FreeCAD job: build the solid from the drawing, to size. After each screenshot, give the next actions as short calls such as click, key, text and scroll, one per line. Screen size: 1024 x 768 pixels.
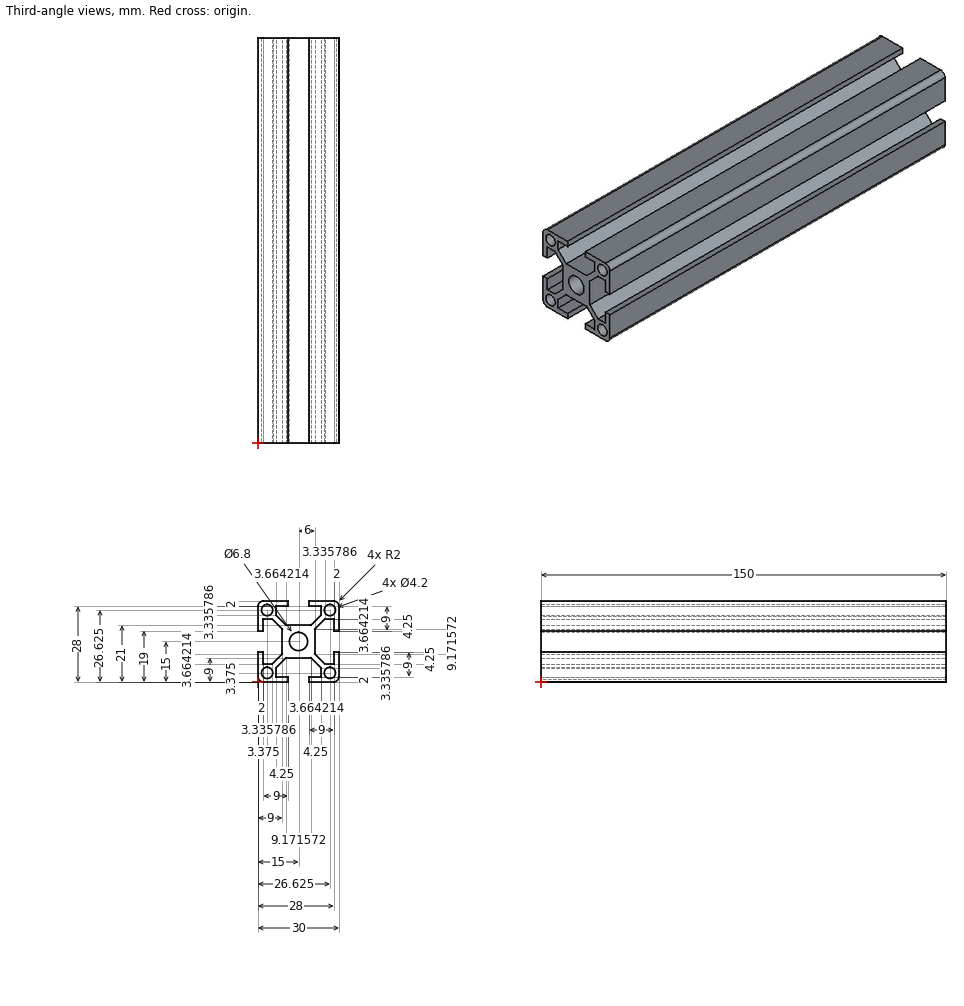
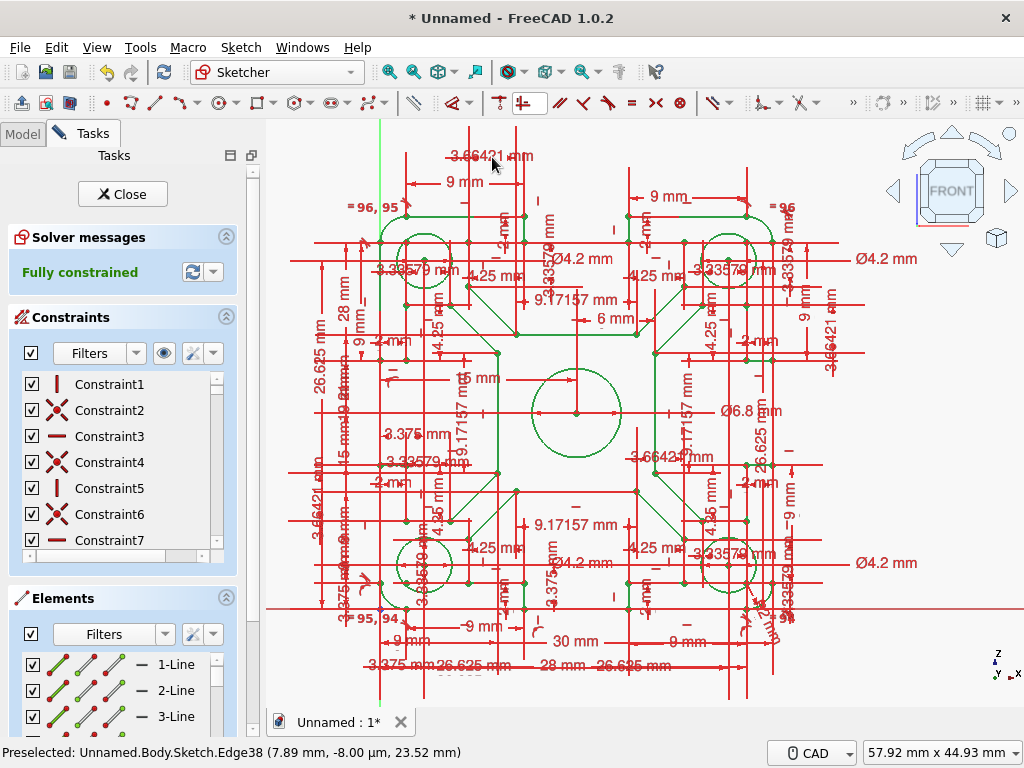
click(123, 194)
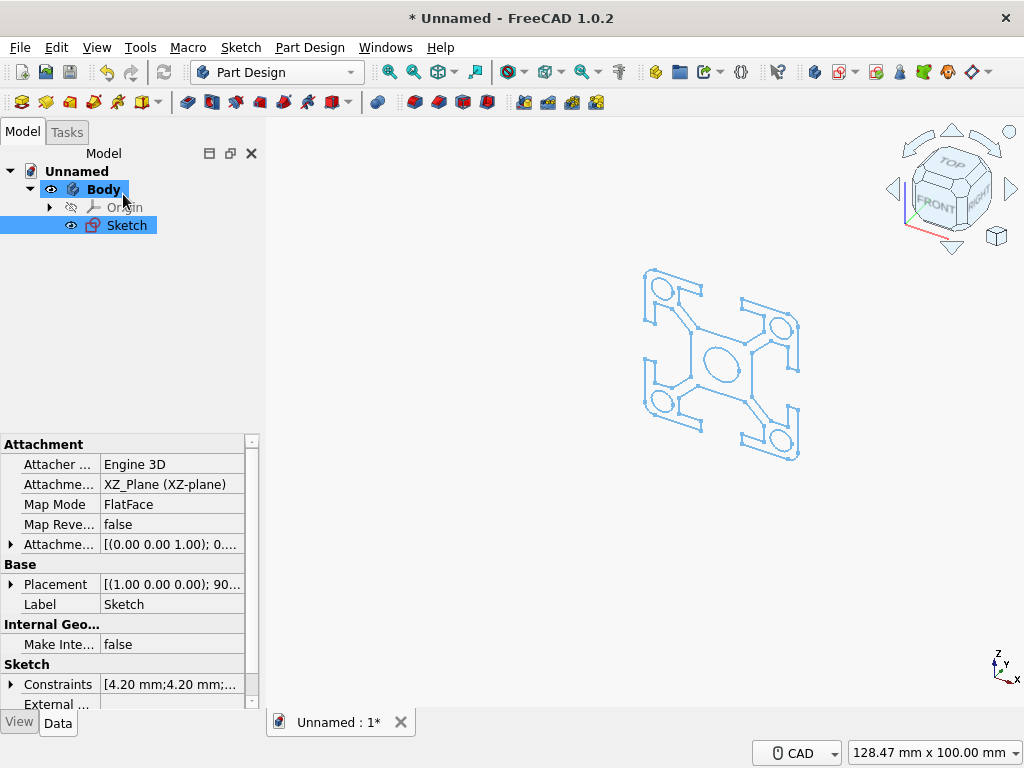
click(22, 102)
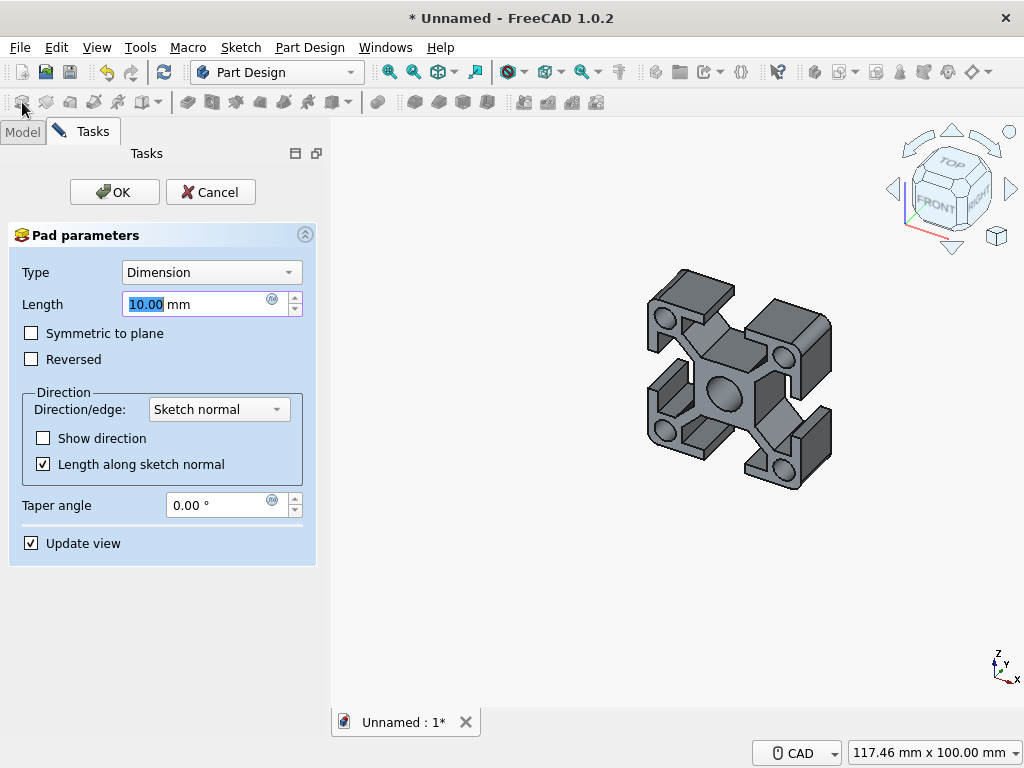
text(150)
key(Tab)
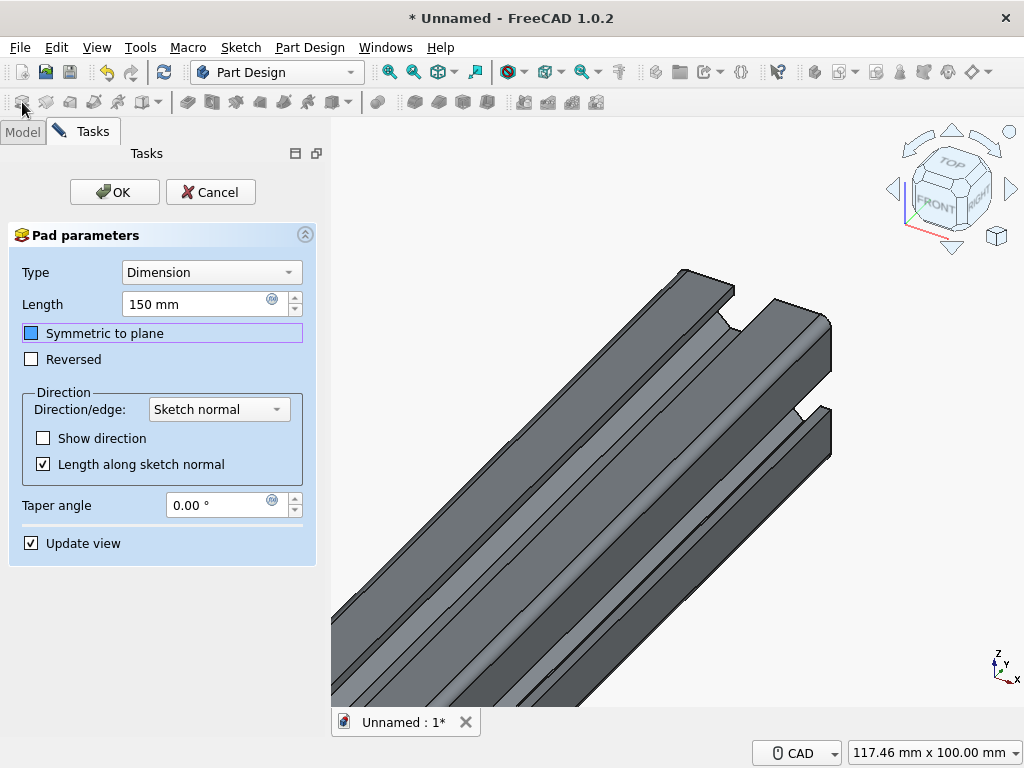
click(30, 359)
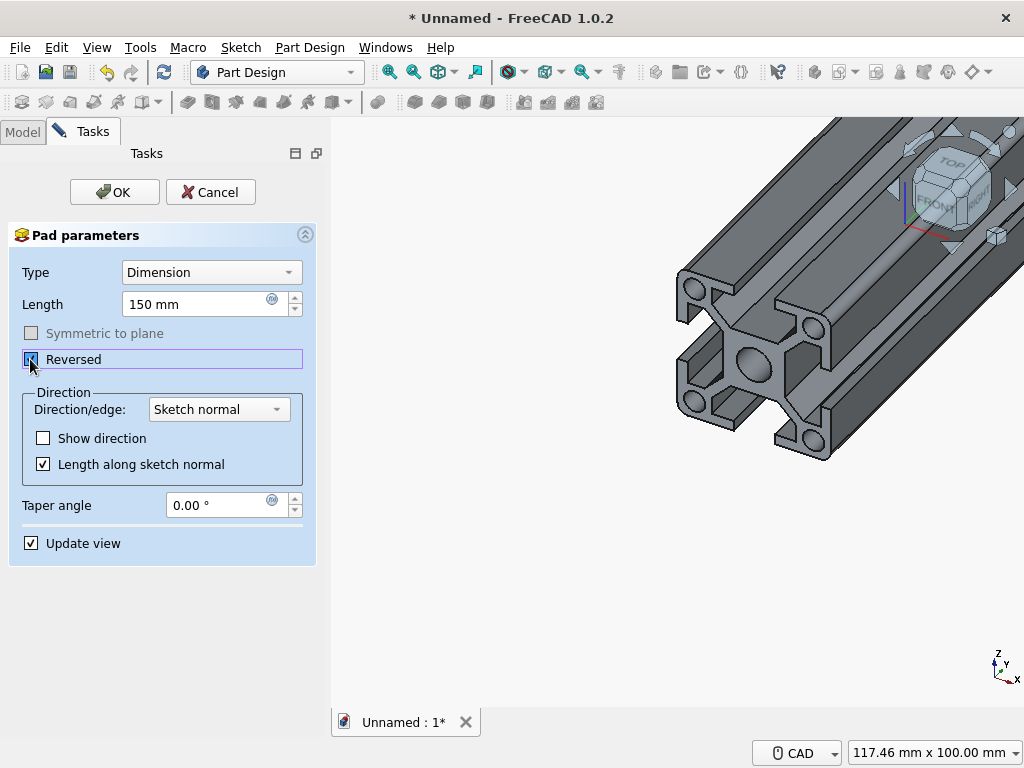
click(115, 192)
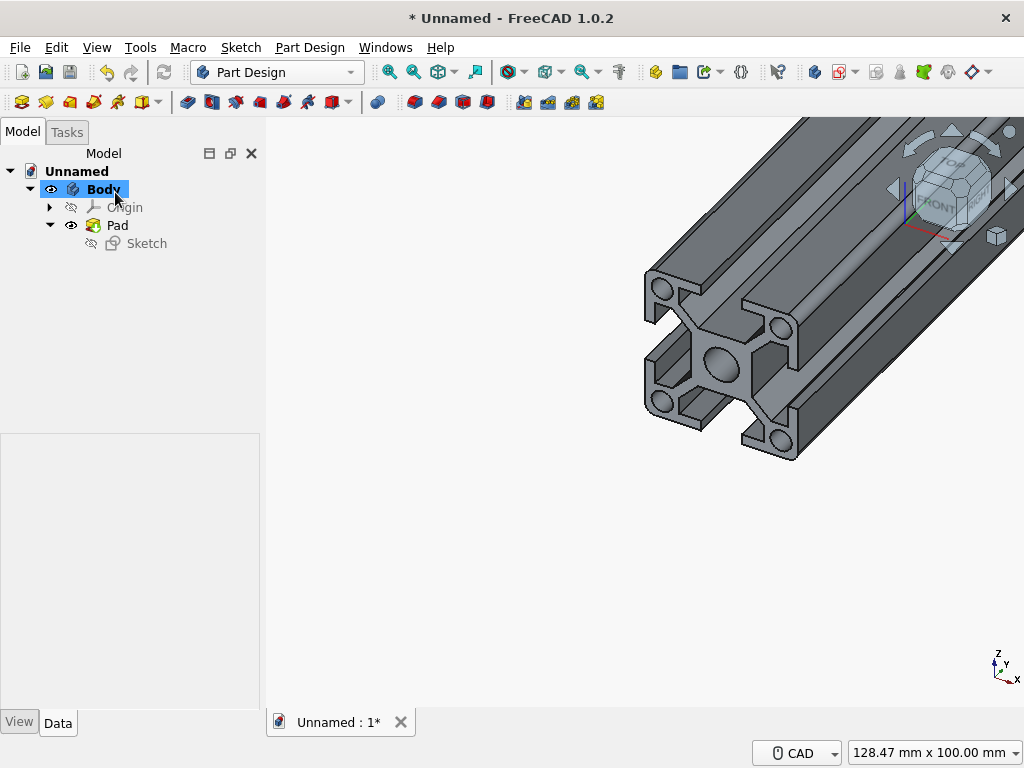
key(0)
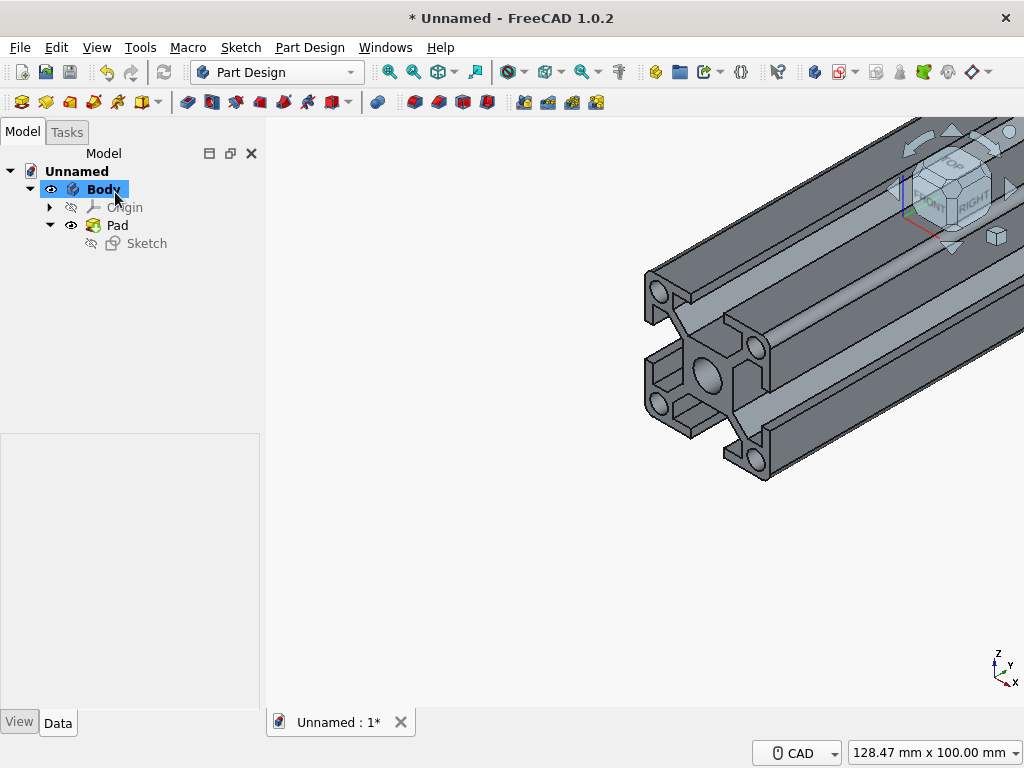
key(v)
key(f)